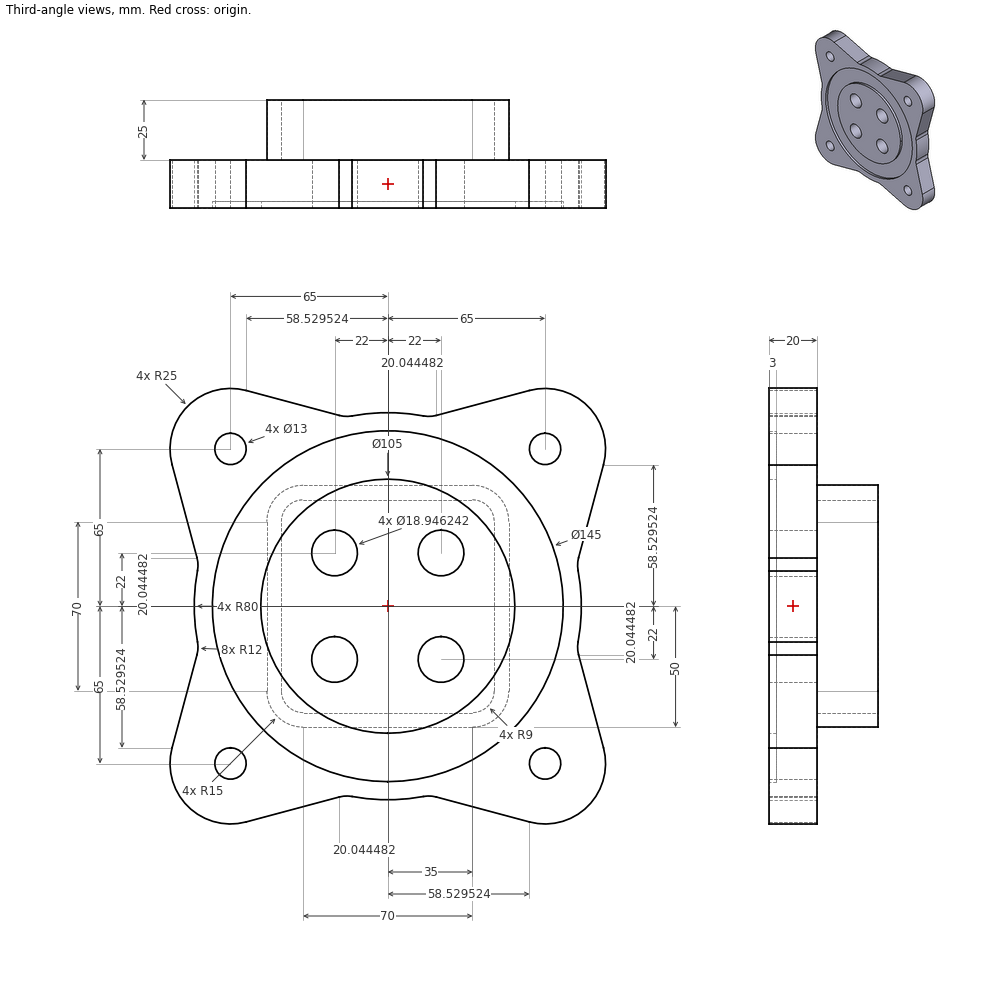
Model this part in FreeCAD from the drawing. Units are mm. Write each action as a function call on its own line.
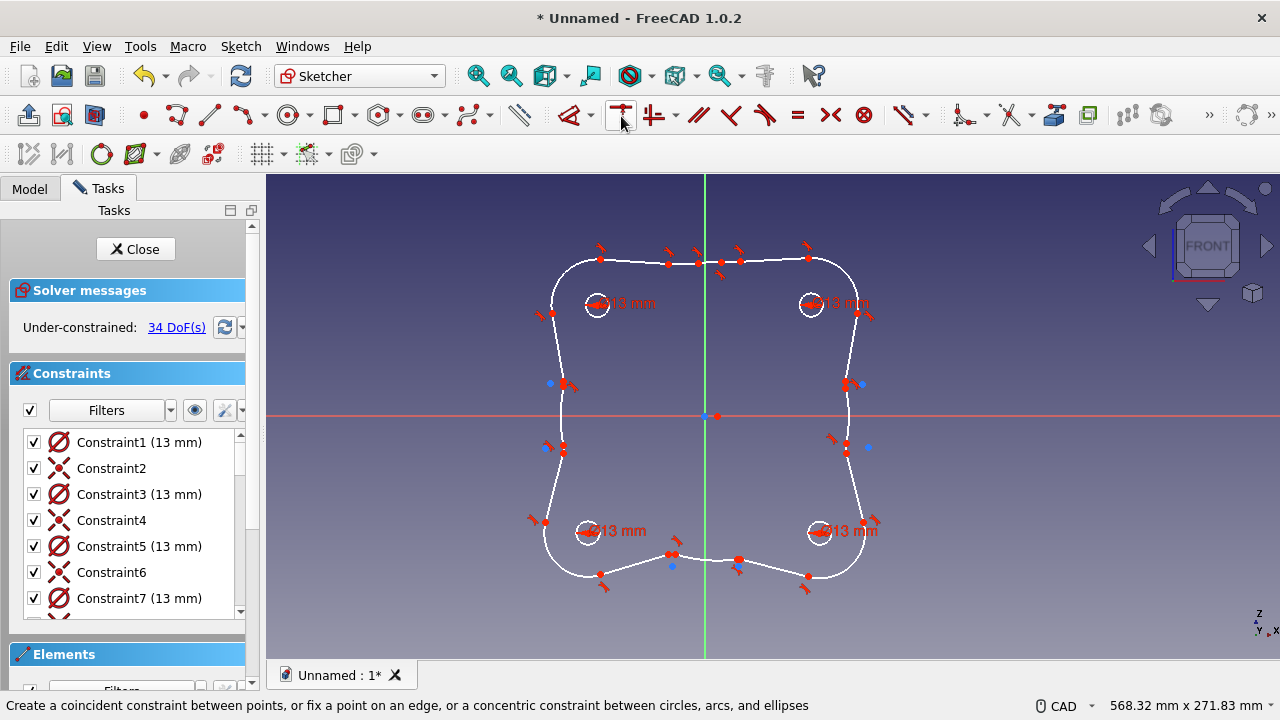
scroll(711, 417, up, 9)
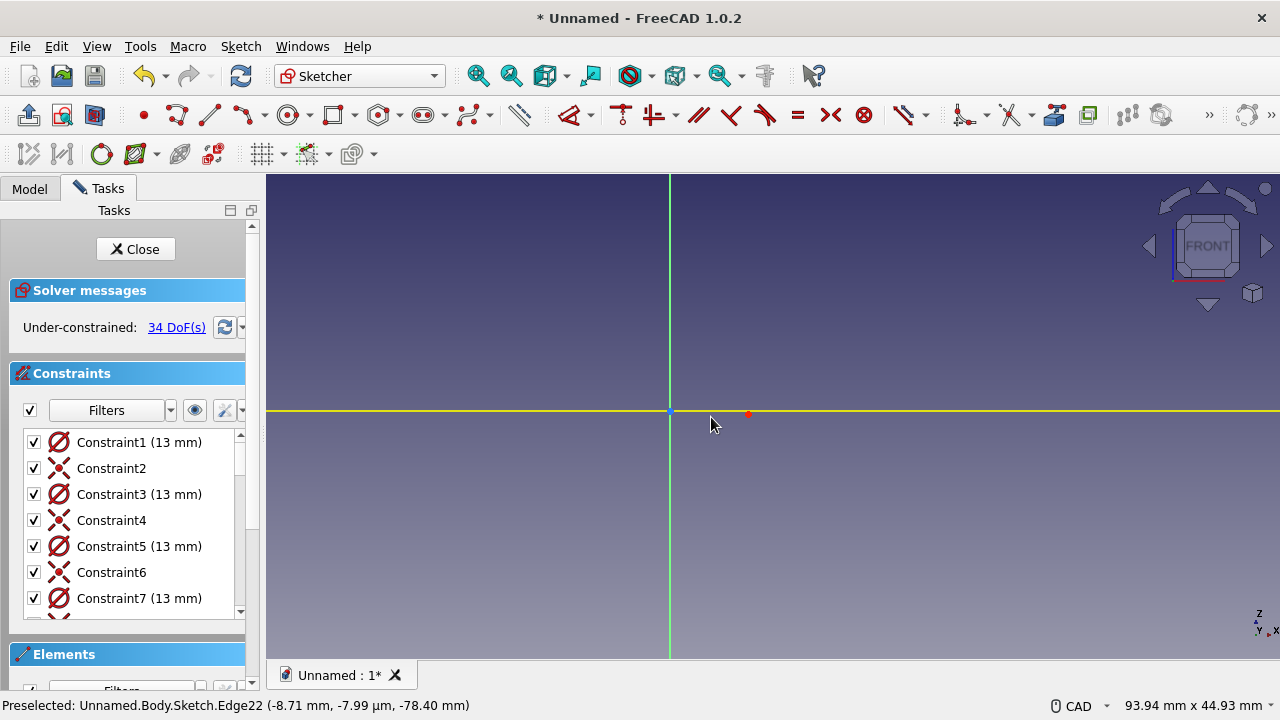
drag(660, 401, 758, 424)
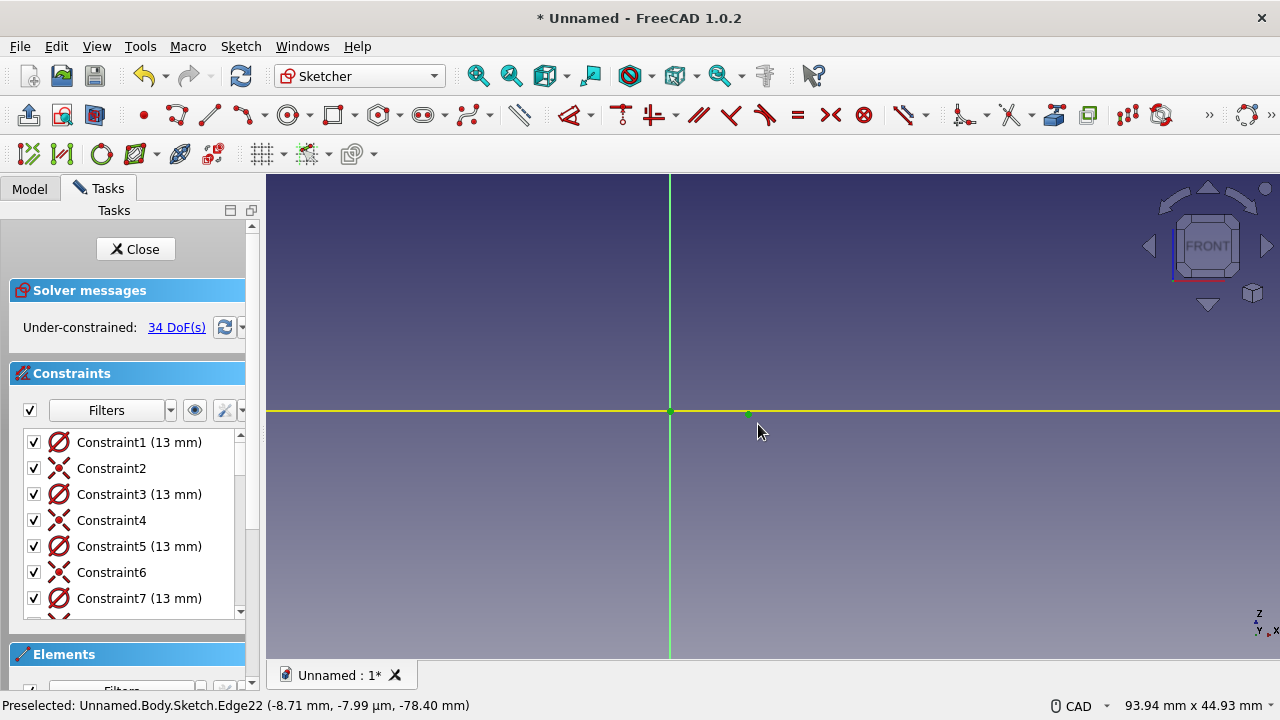
key(c)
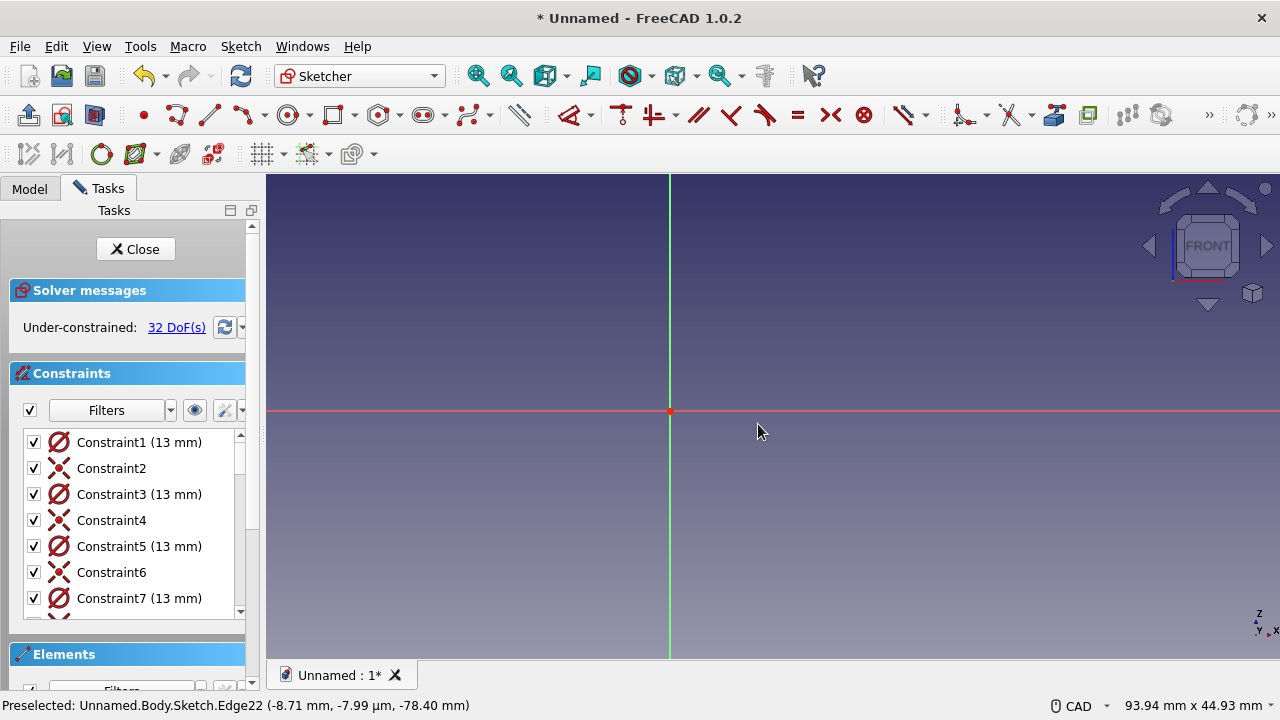
scroll(711, 418, down, 9)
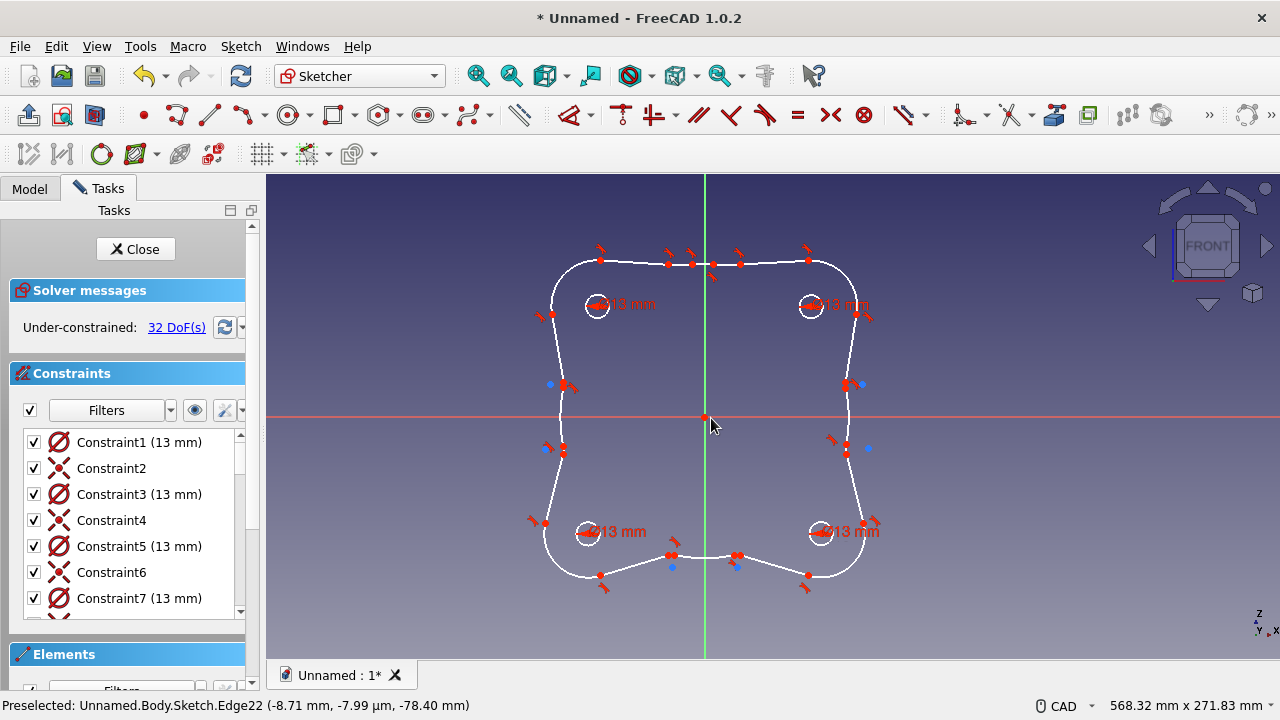
scroll(564, 452, up, 9)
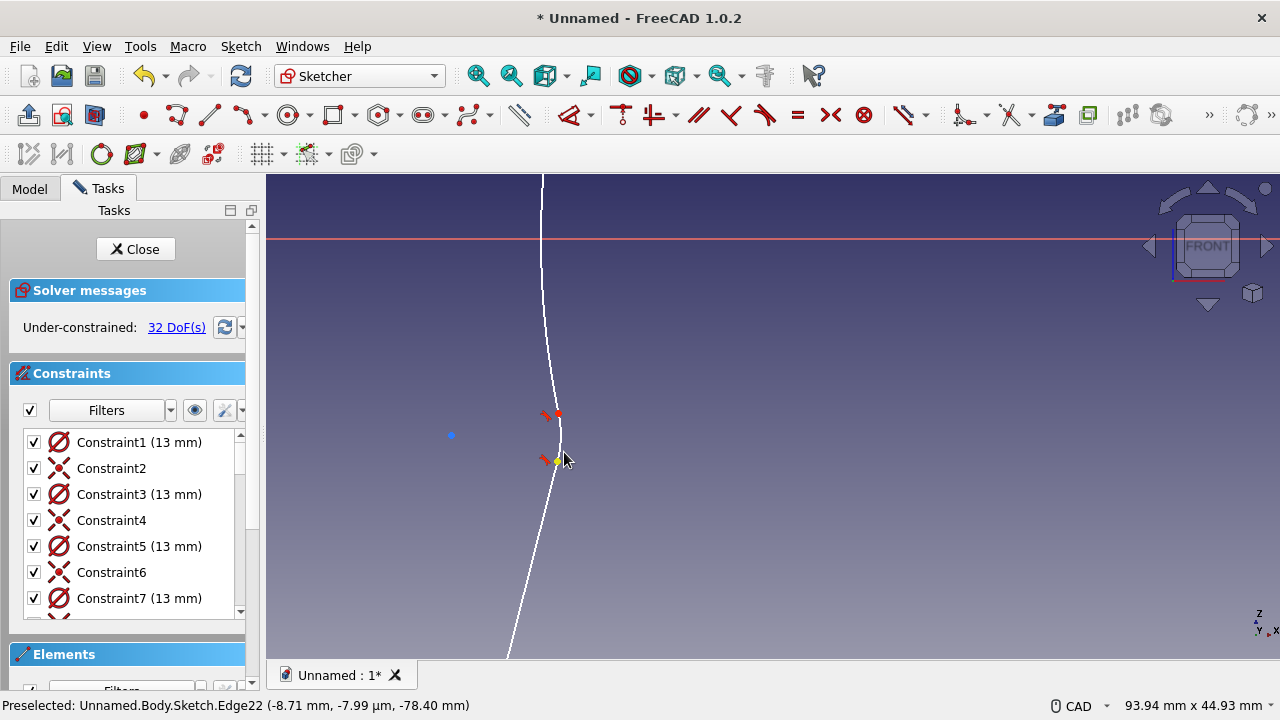
click(560, 447)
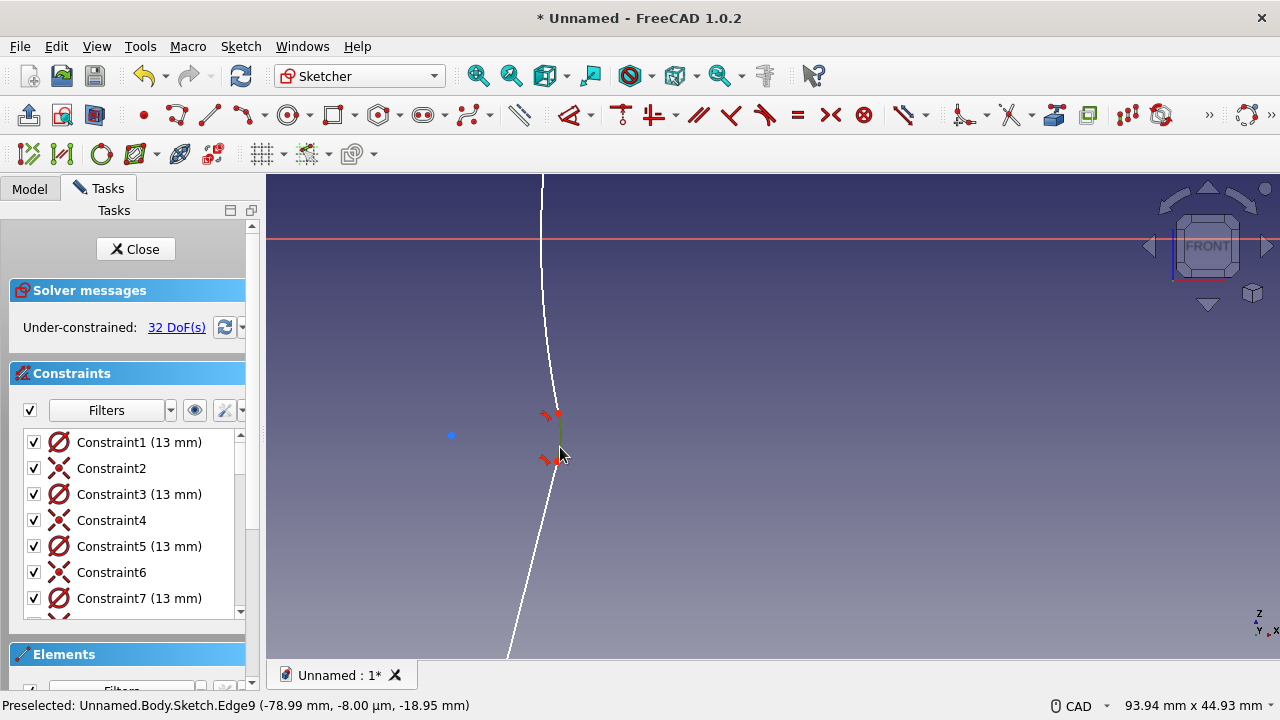
scroll(564, 452, down, 9)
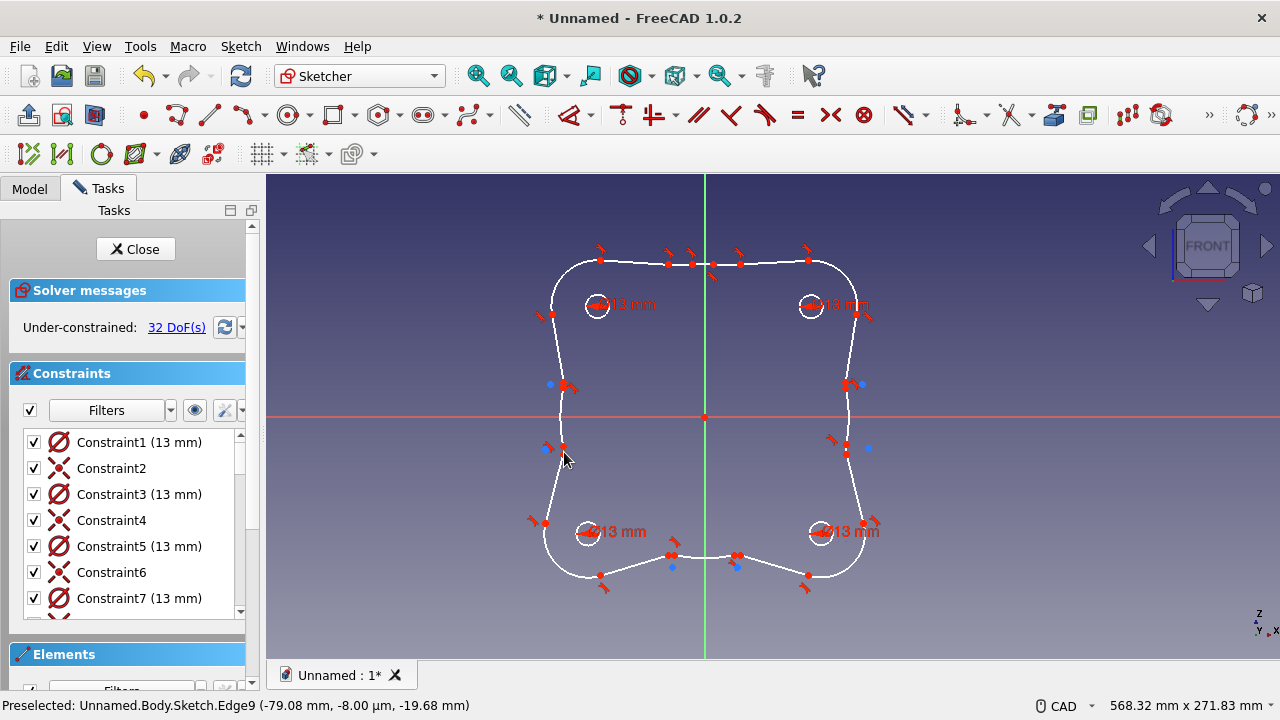
scroll(564, 386, up, 11)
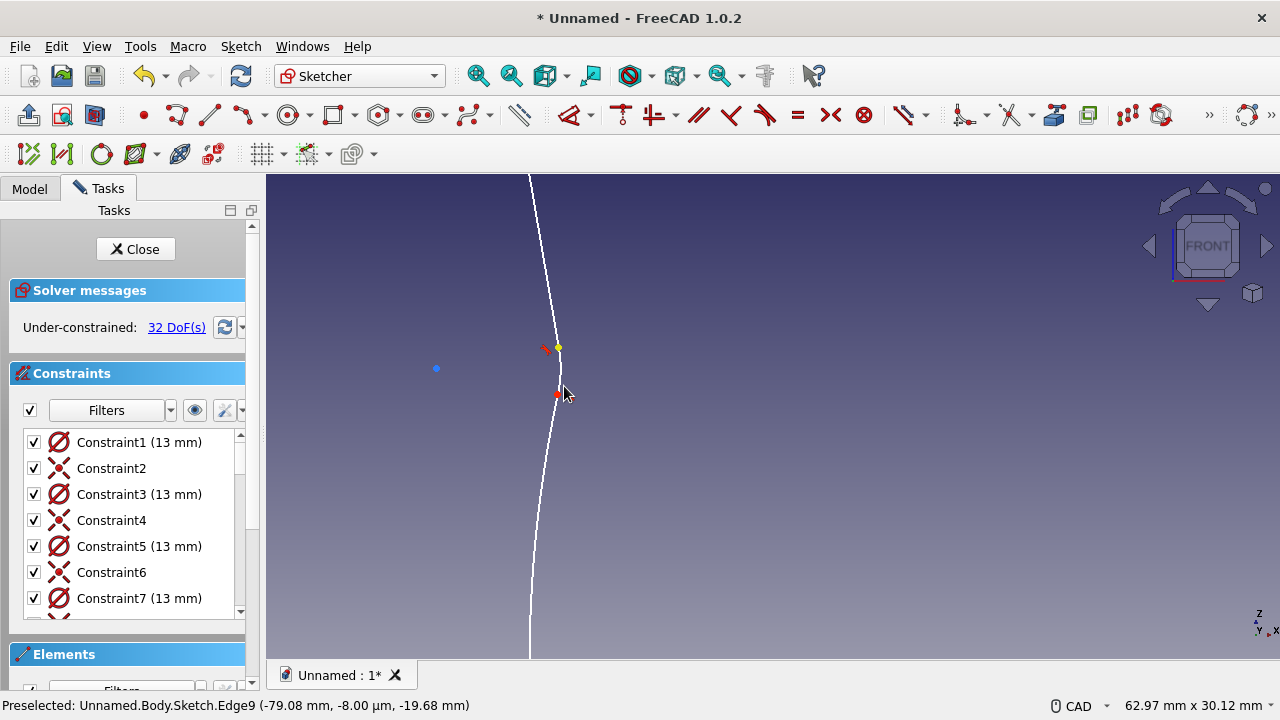
click(560, 380)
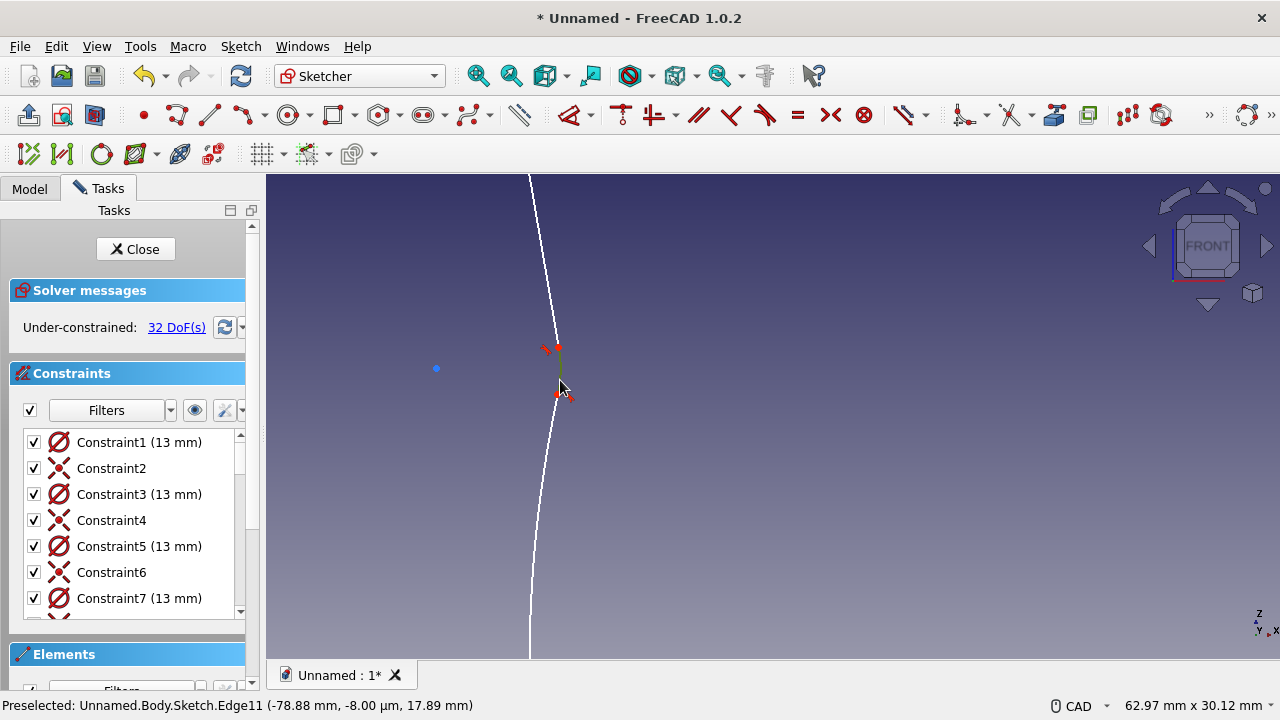
scroll(564, 386, down, 11)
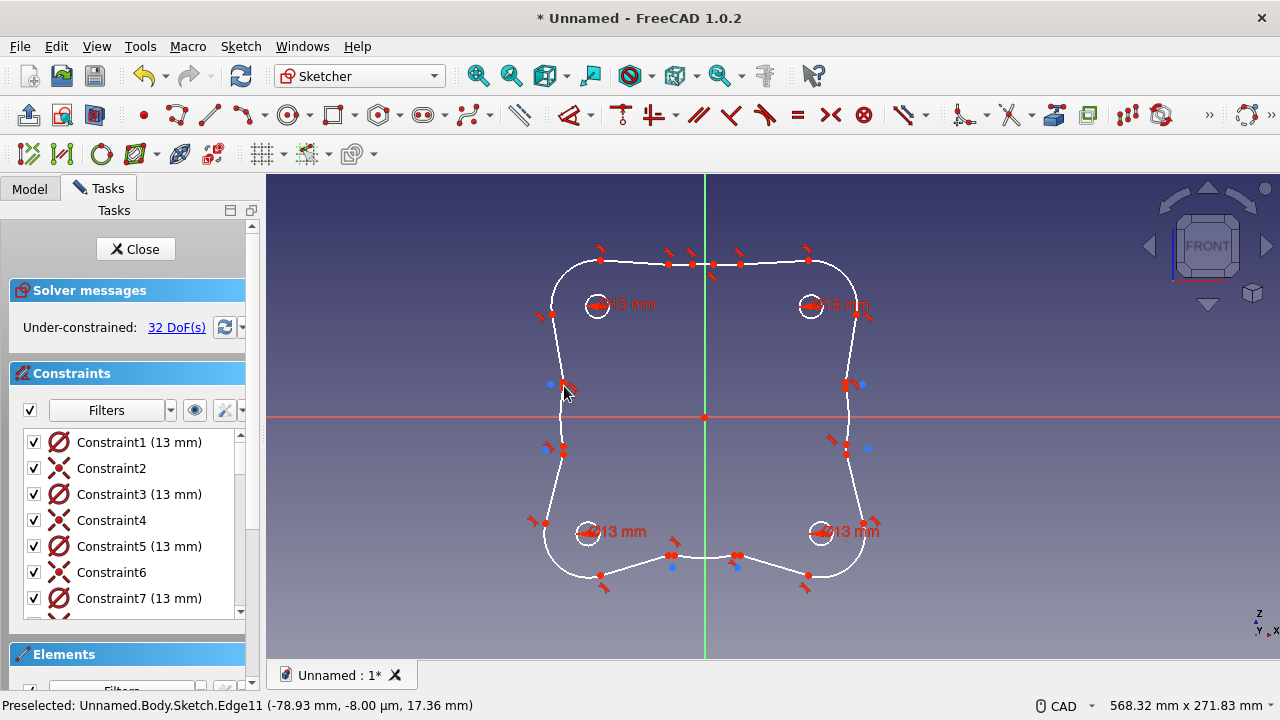
scroll(676, 265, up, 4)